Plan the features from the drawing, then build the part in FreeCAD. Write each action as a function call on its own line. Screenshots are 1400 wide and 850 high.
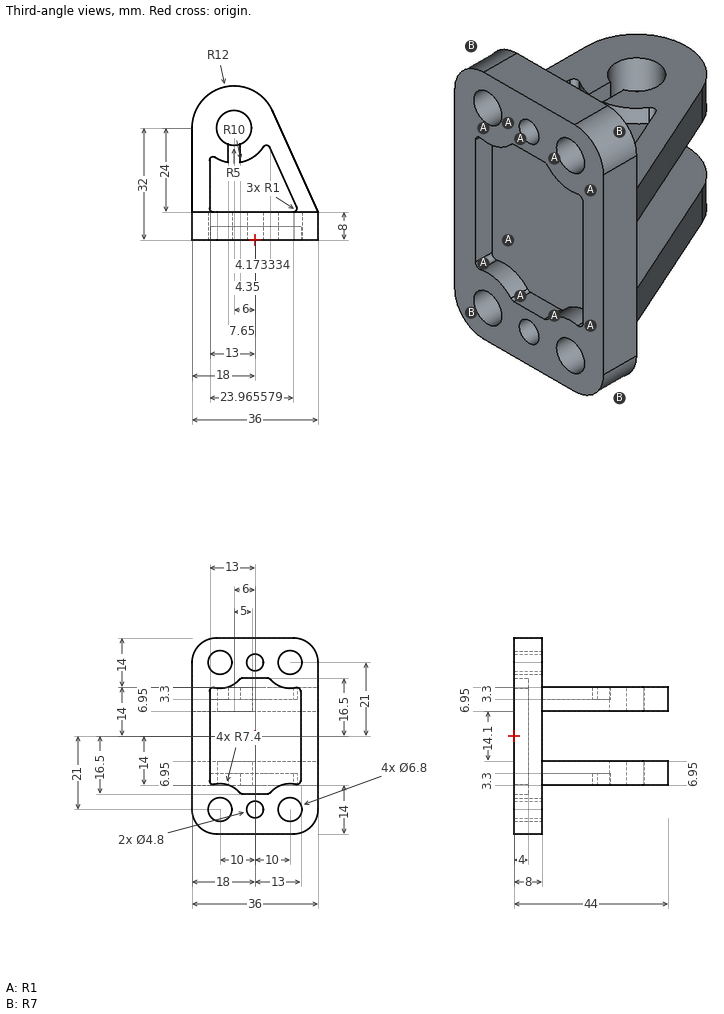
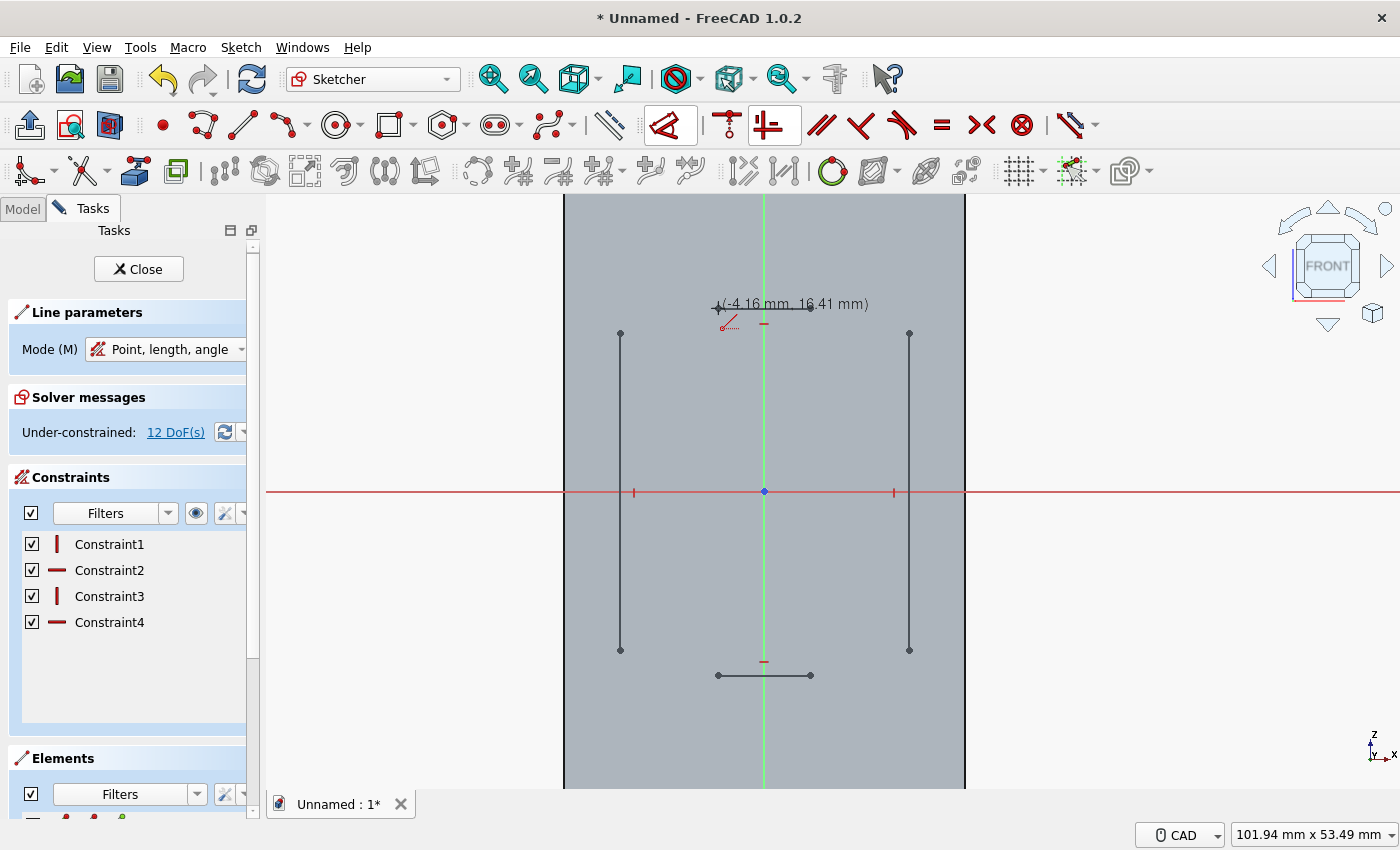
key(g)
key(3)
key(a)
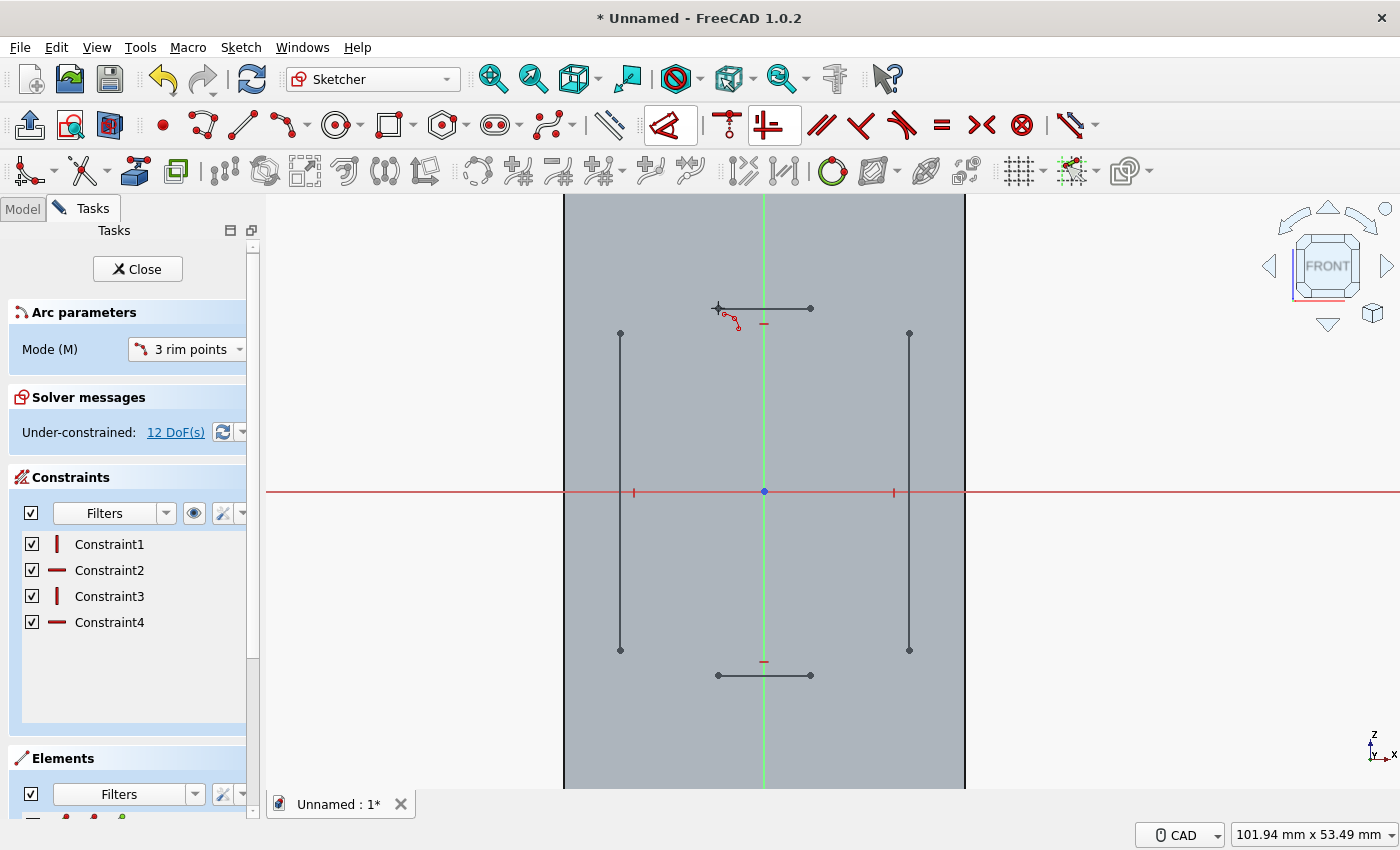
click(620, 651)
click(718, 676)
click(673, 645)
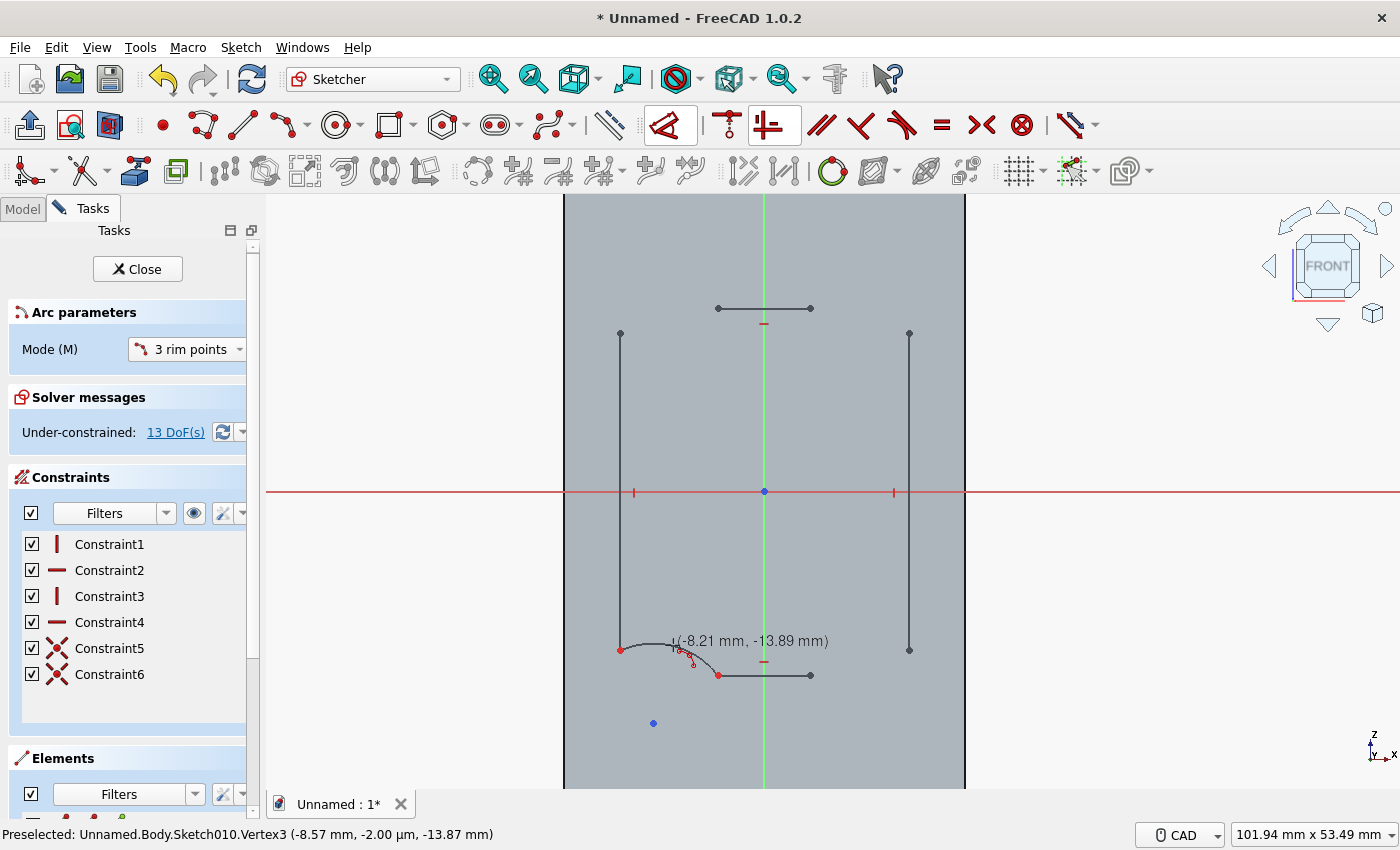
click(810, 676)
click(909, 651)
click(855, 645)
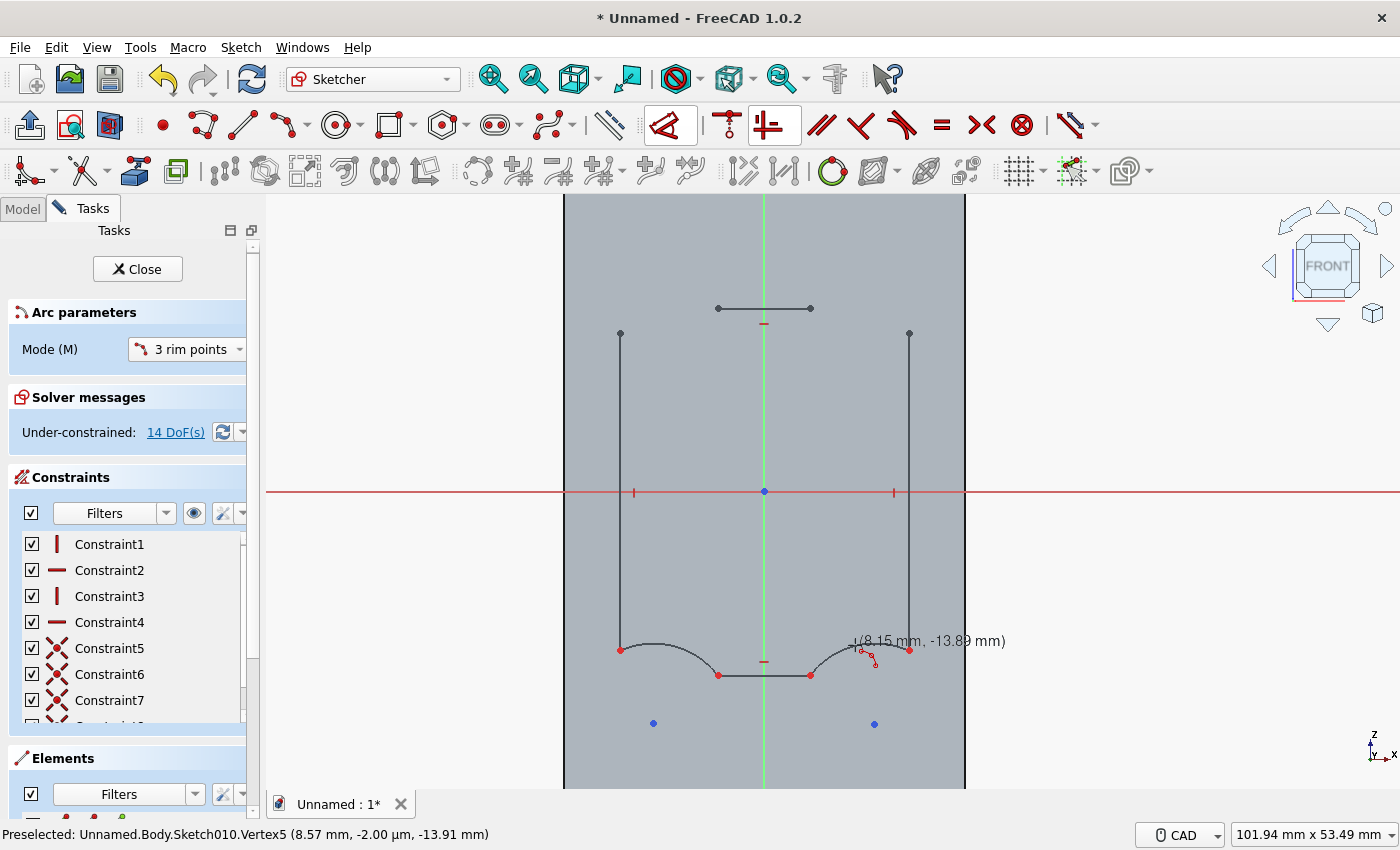
click(909, 334)
click(810, 309)
click(855, 338)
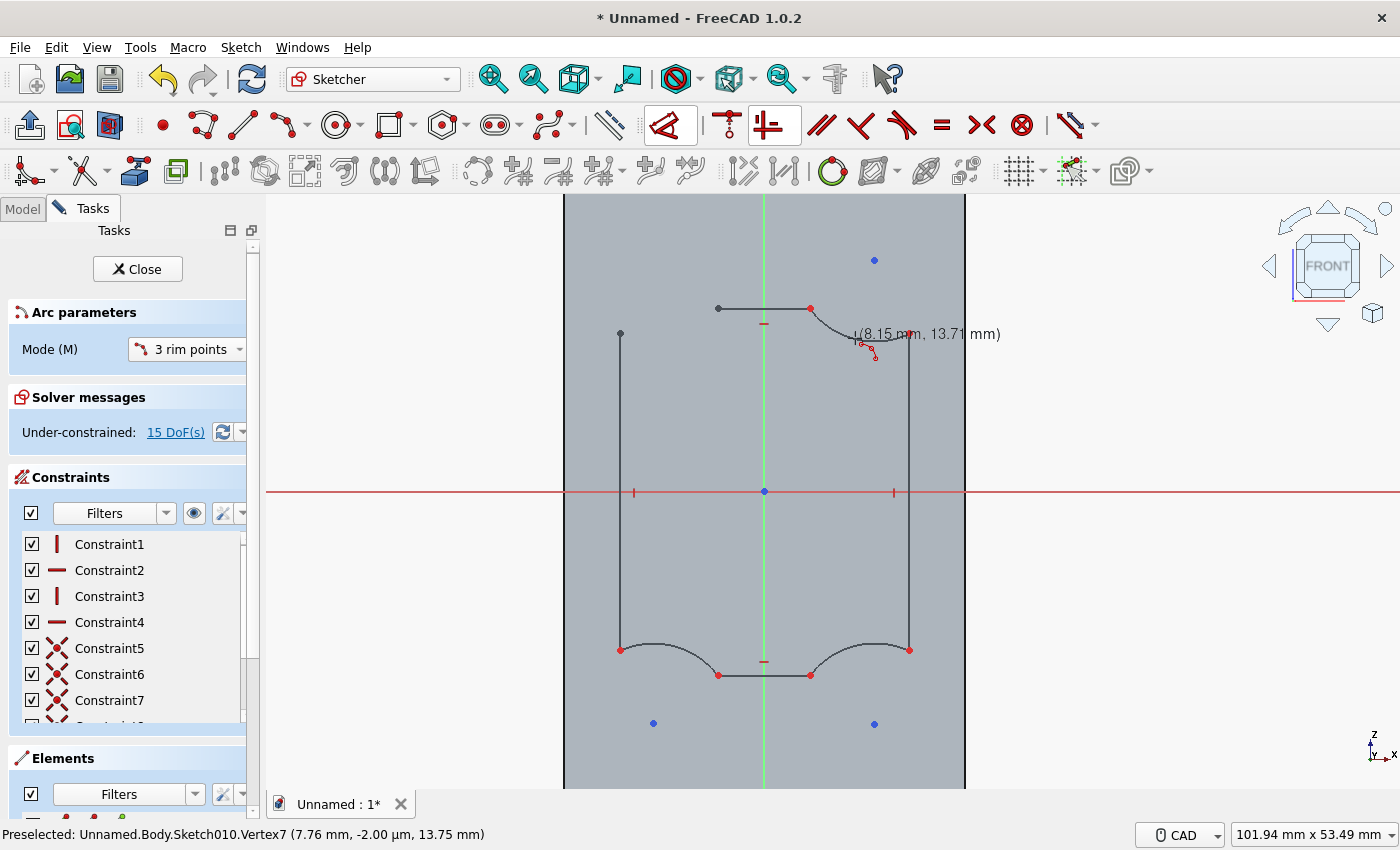
click(718, 309)
click(620, 334)
click(673, 338)
key(Escape)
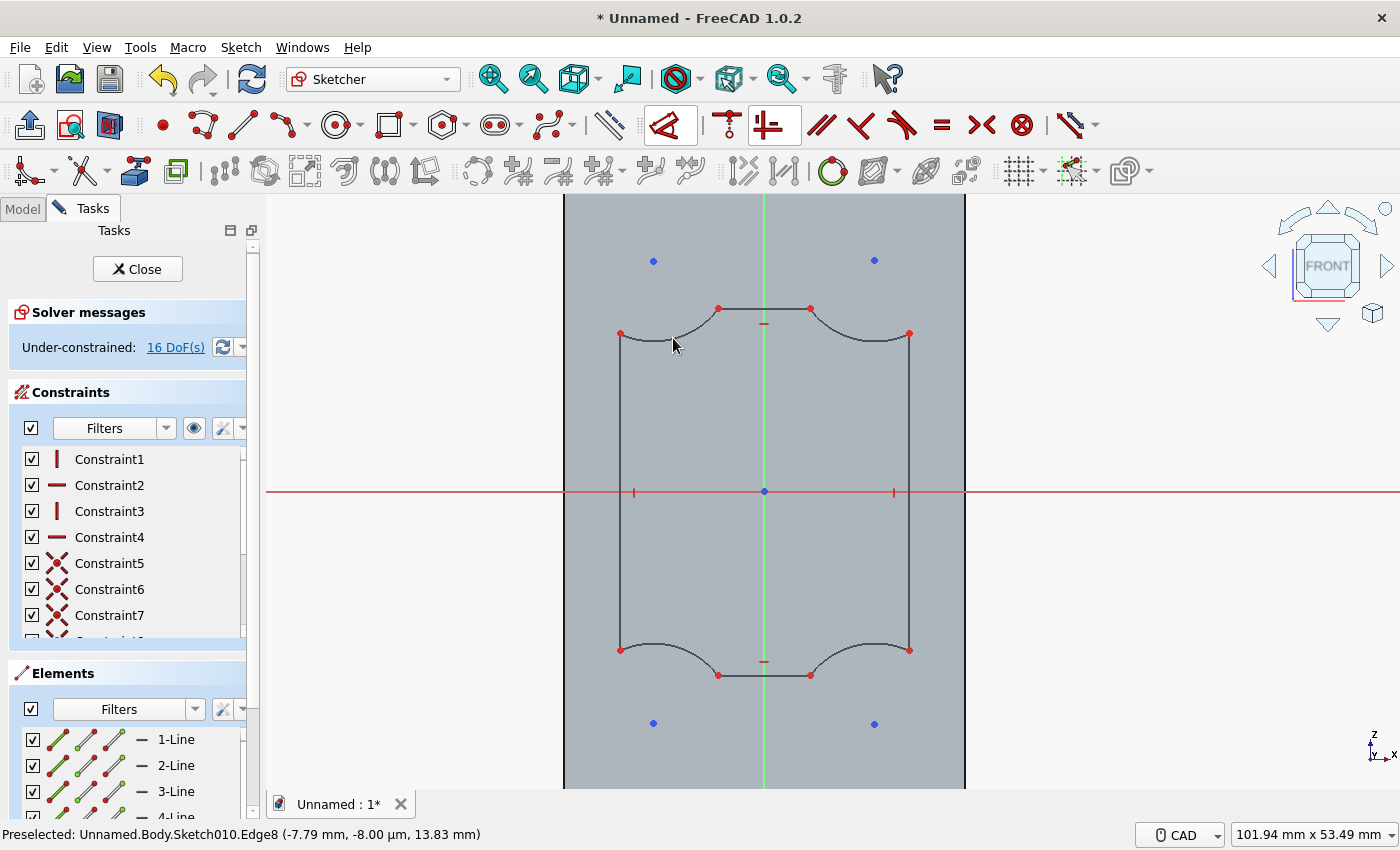
click(694, 654)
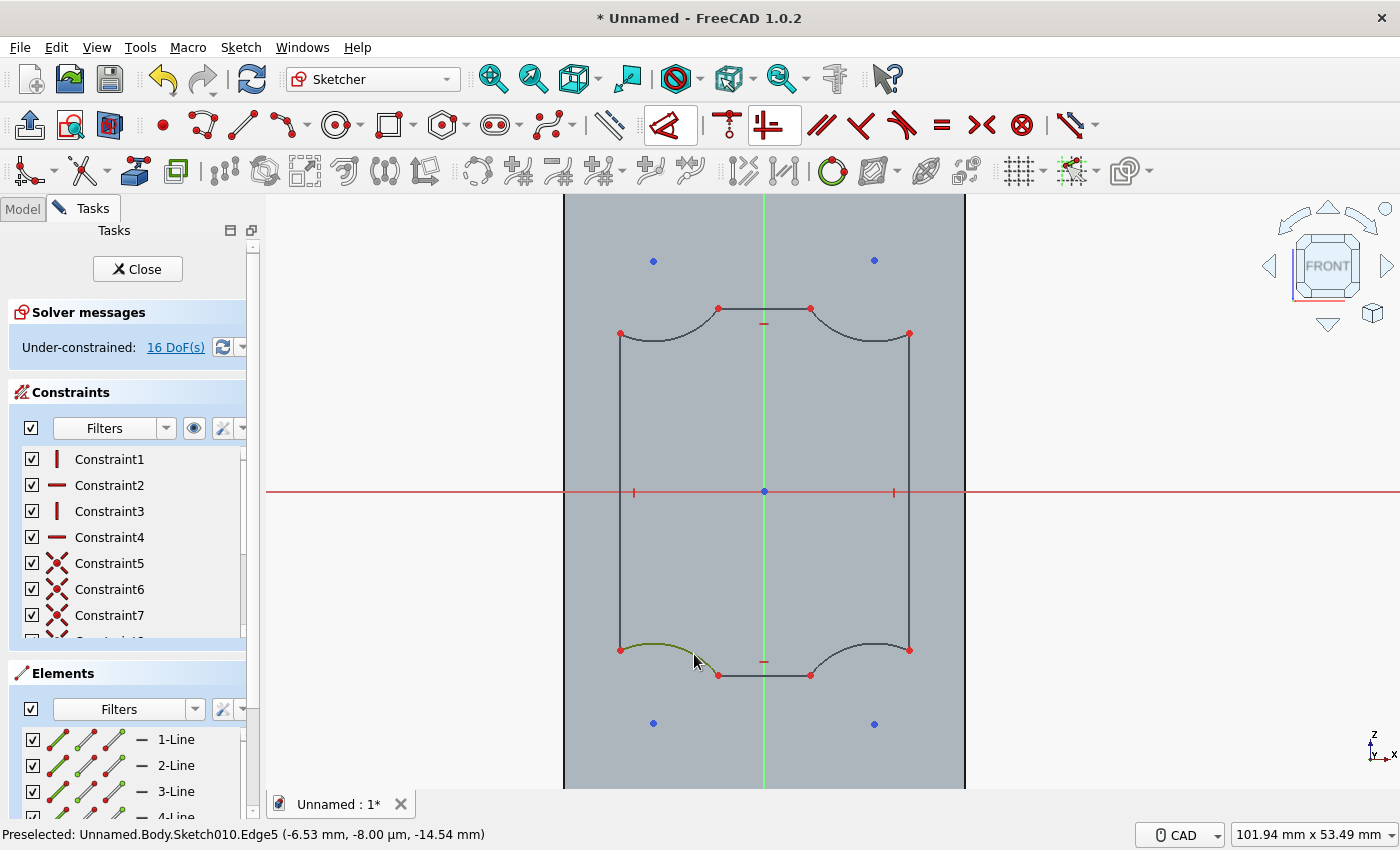
click(877, 644)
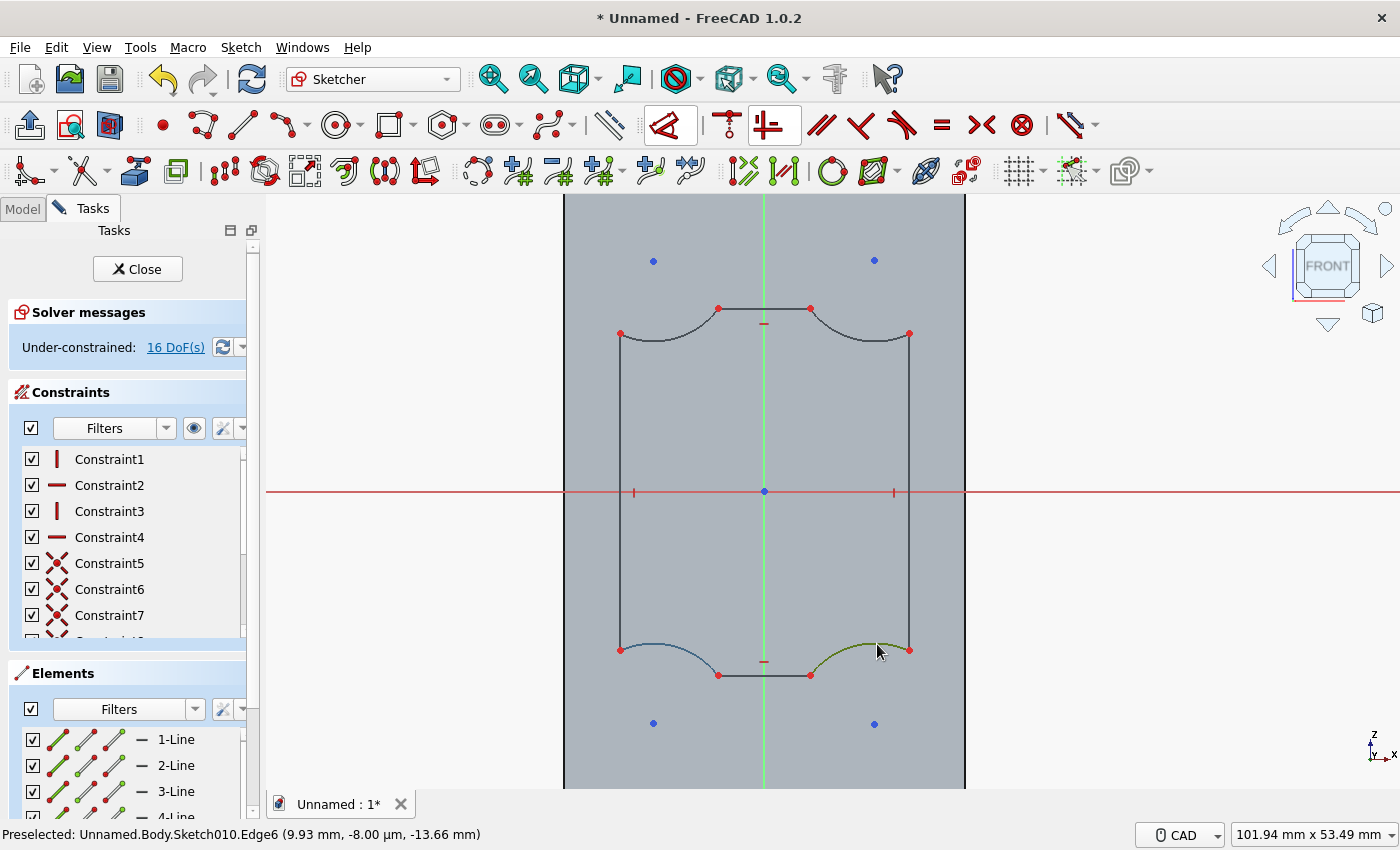
click(835, 331)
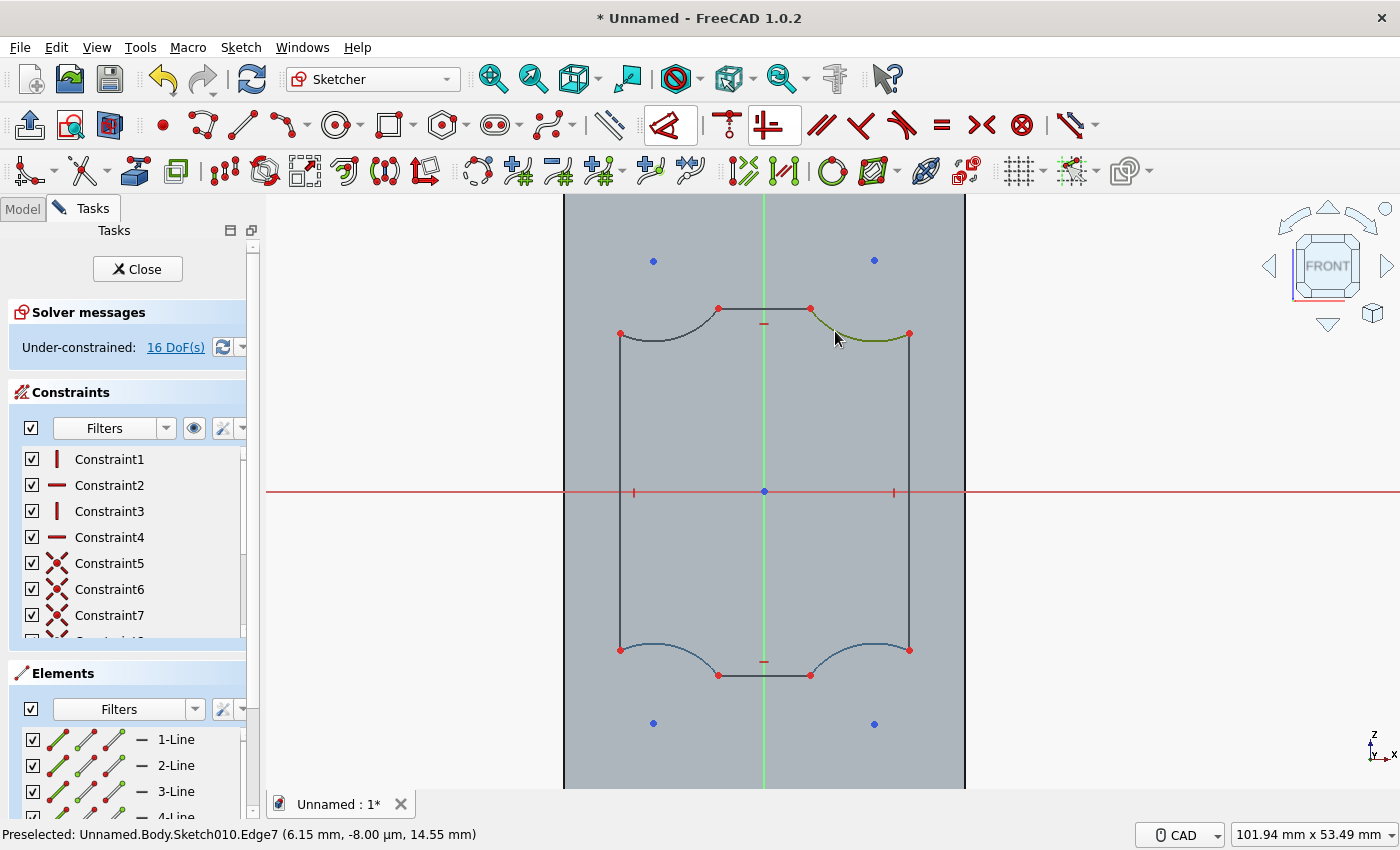
click(652, 341)